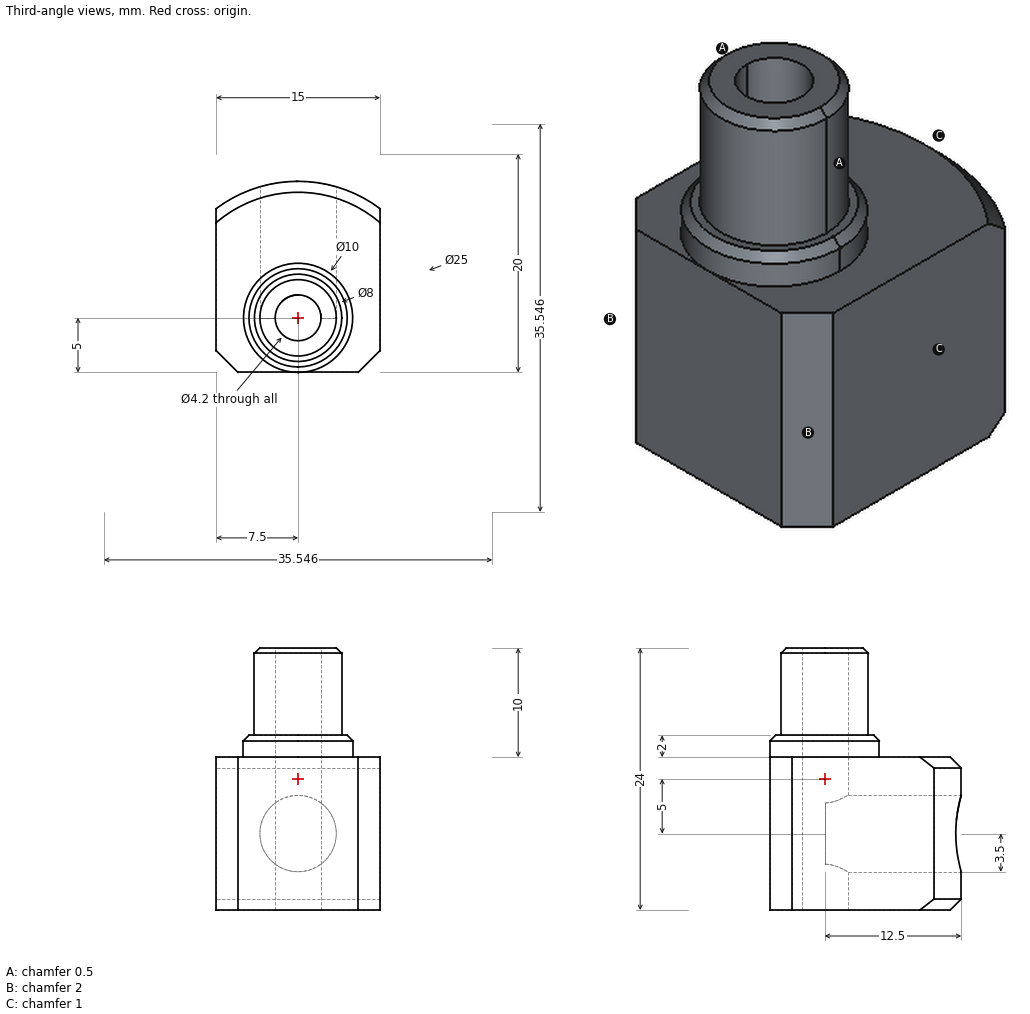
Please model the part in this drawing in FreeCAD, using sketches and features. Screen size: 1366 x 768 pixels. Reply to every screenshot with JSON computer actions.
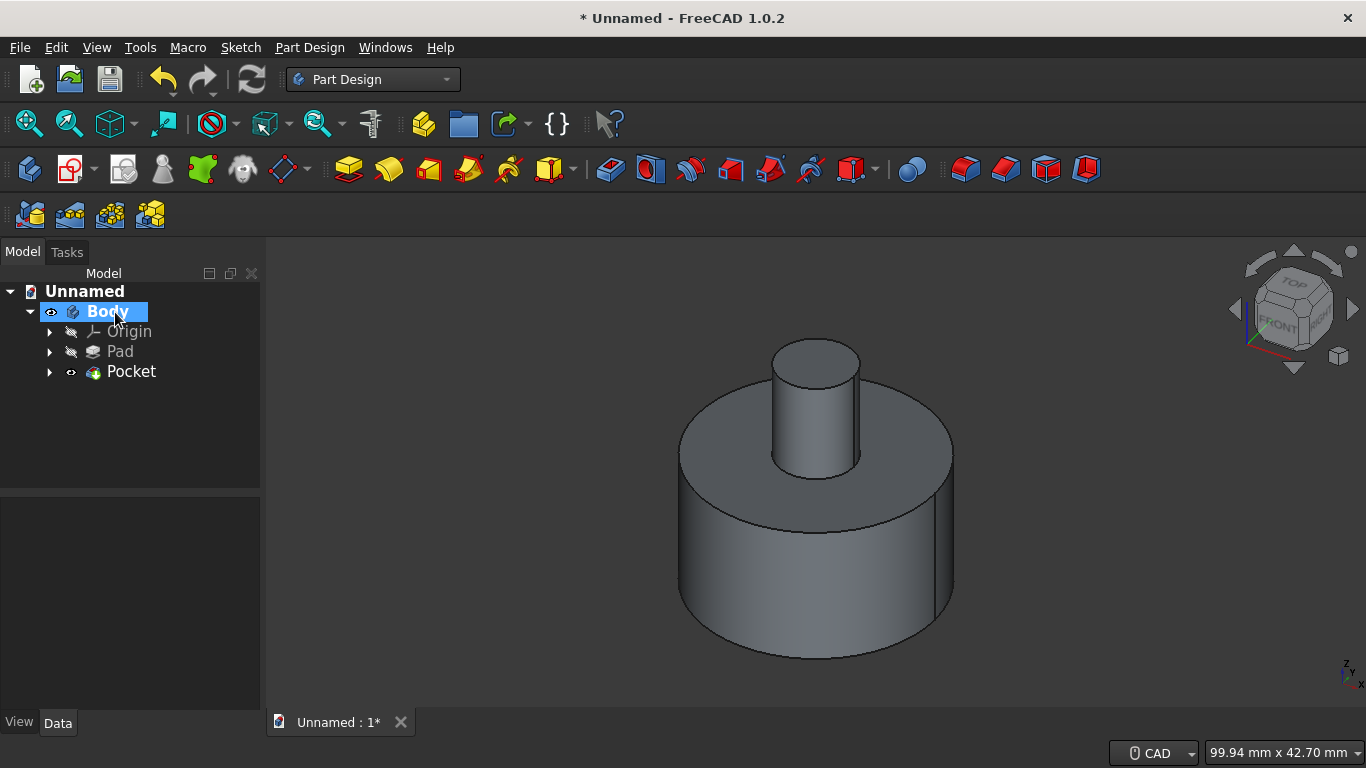
{"action": "key", "text": "5"}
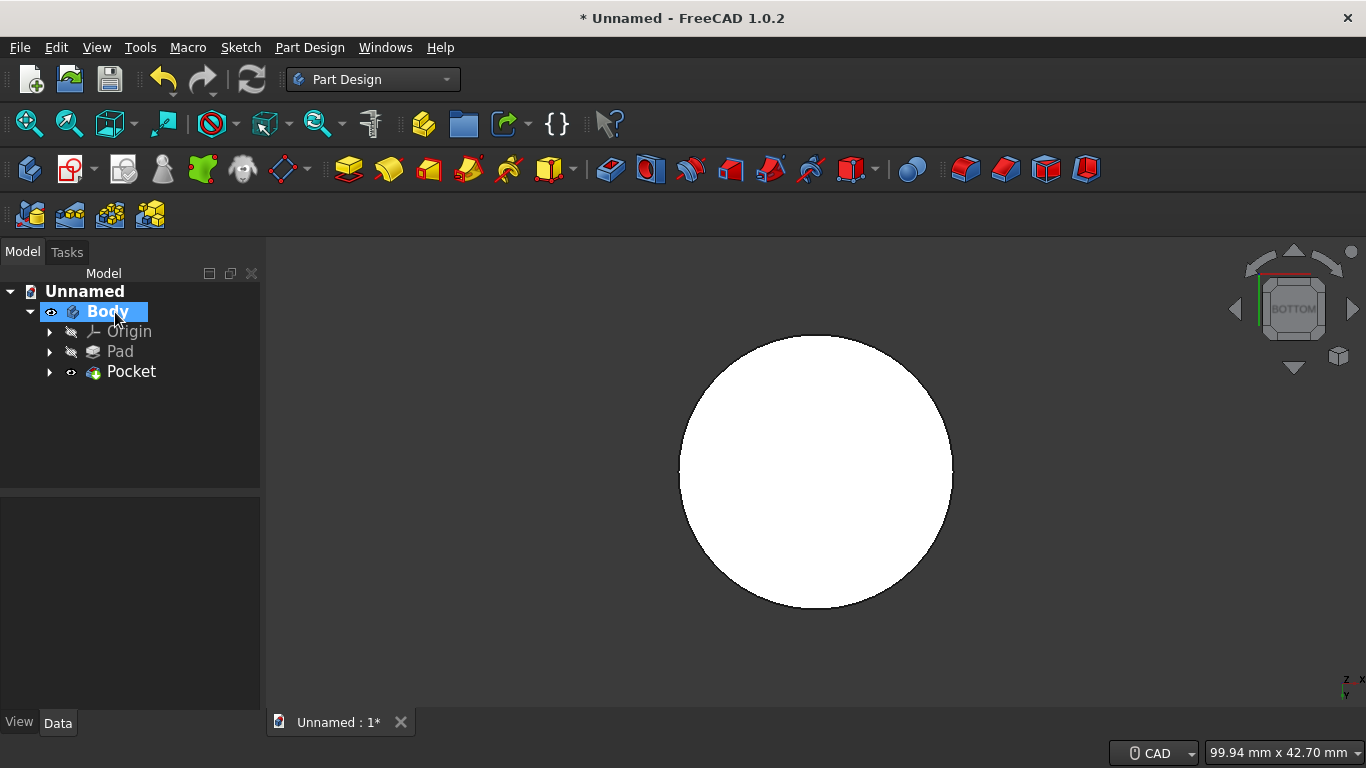
{"action": "left_click", "coordinate": [816, 471]}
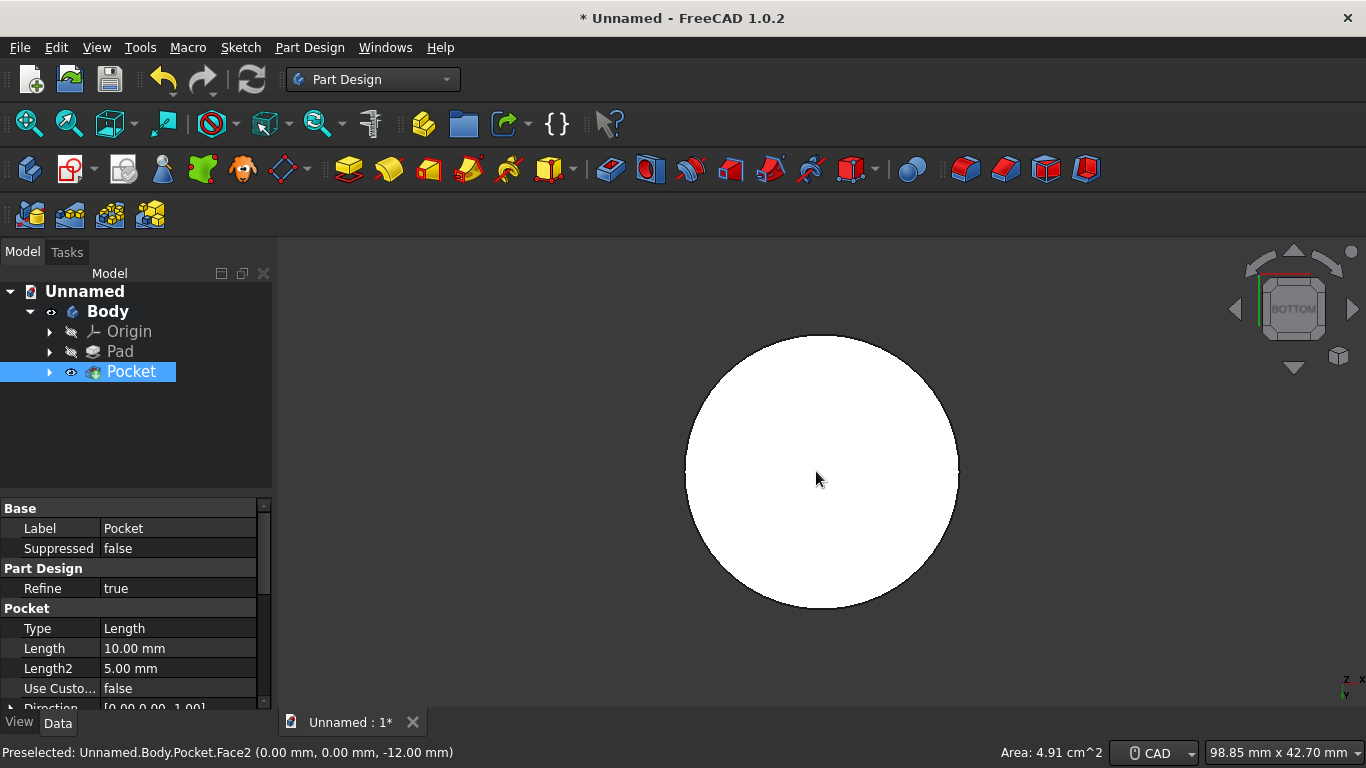
{"action": "left_click", "coordinate": [70, 170]}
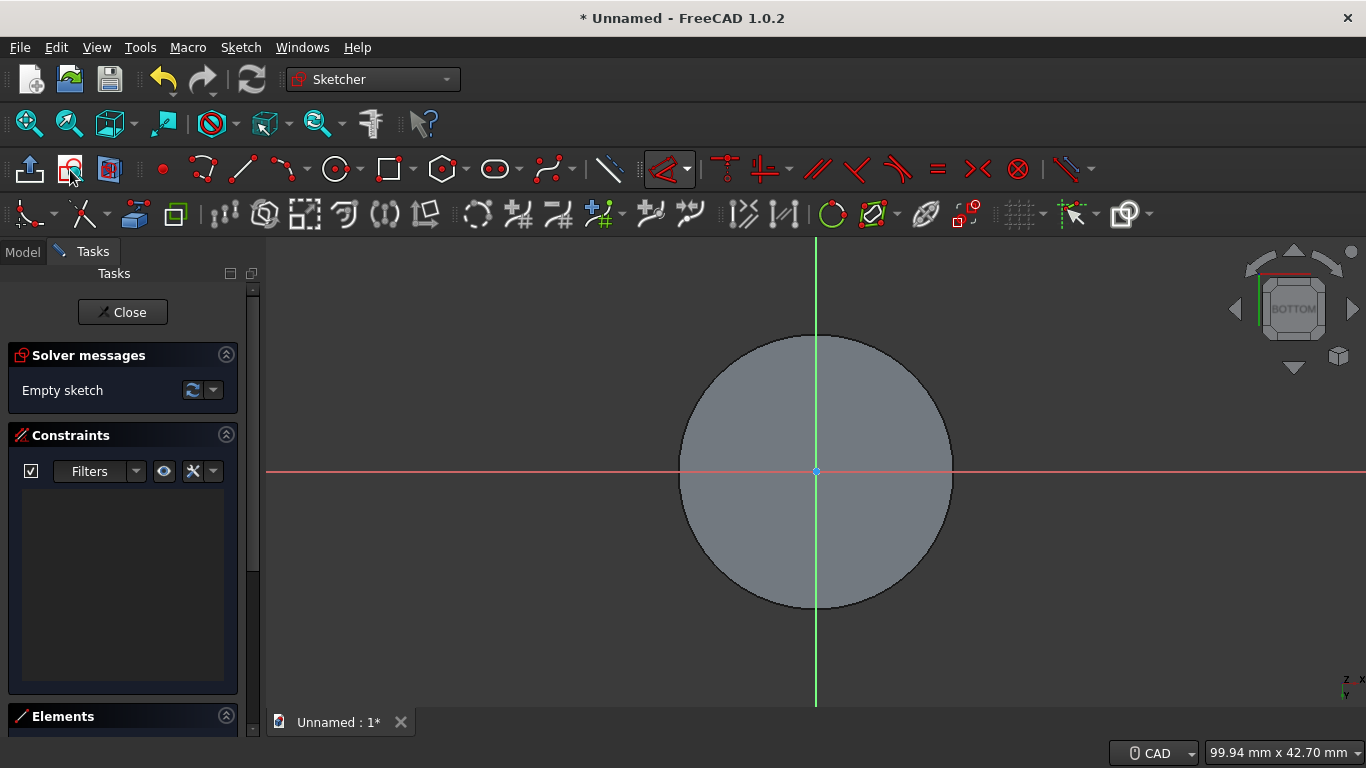
{"action": "scroll", "coordinate": [438, 472], "scroll_direction": "down", "scroll_amount": 1}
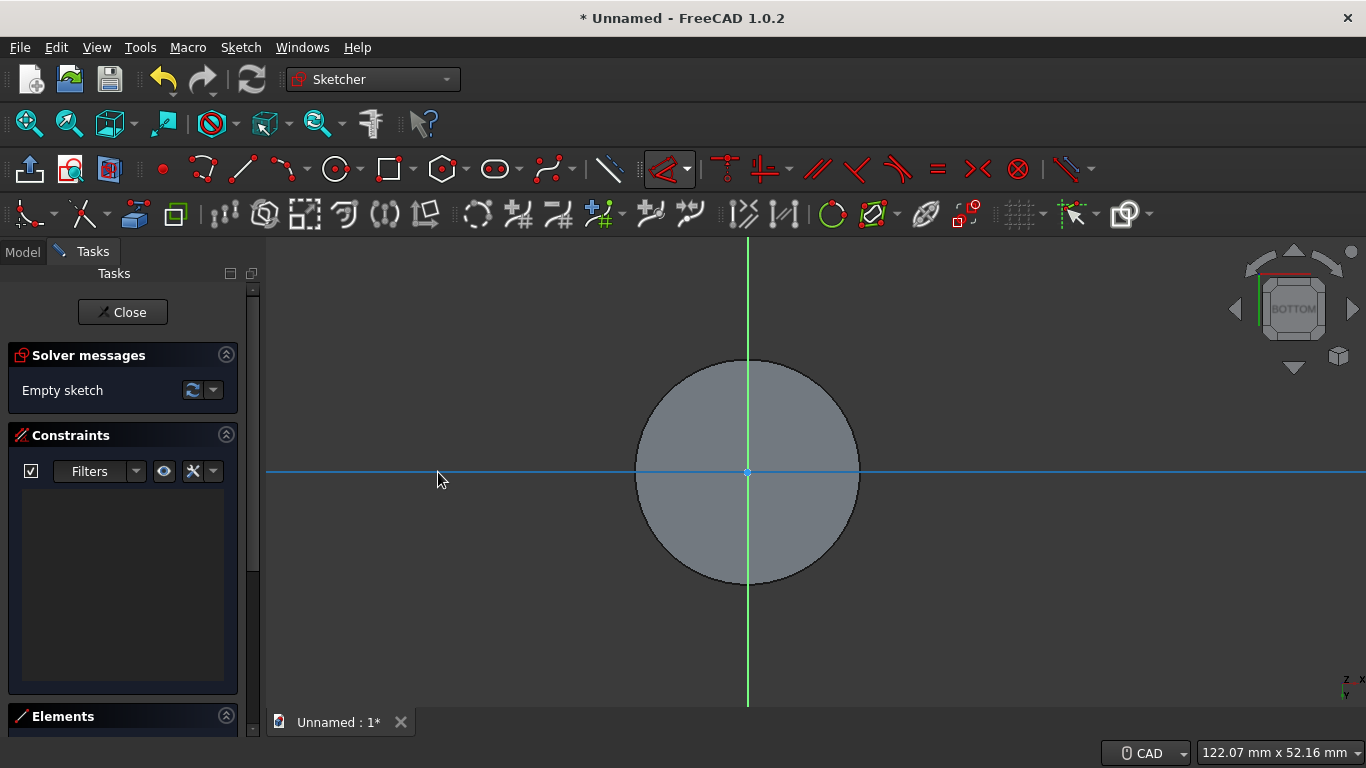
{"action": "key", "text": "g v"}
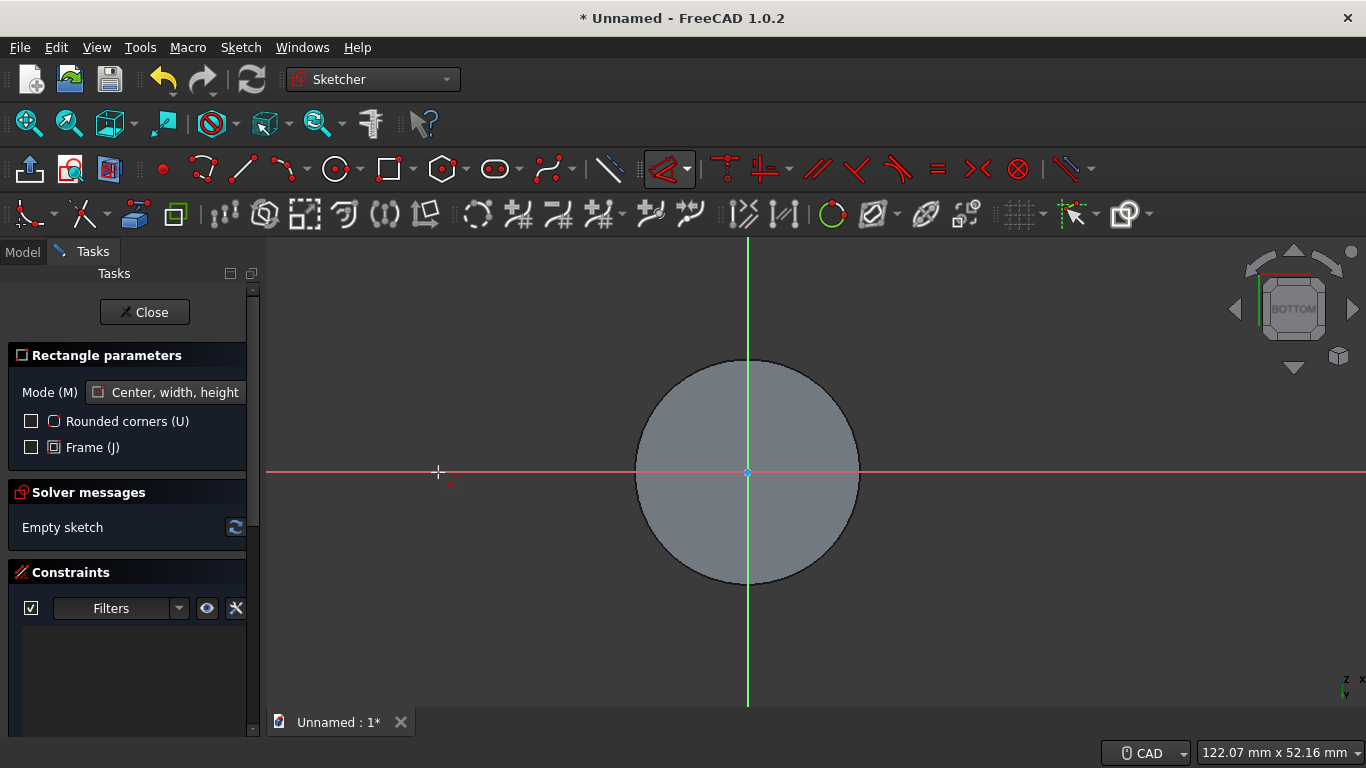
{"action": "left_click", "coordinate": [748, 472]}
{"action": "mouse_move", "coordinate": [908, 312]}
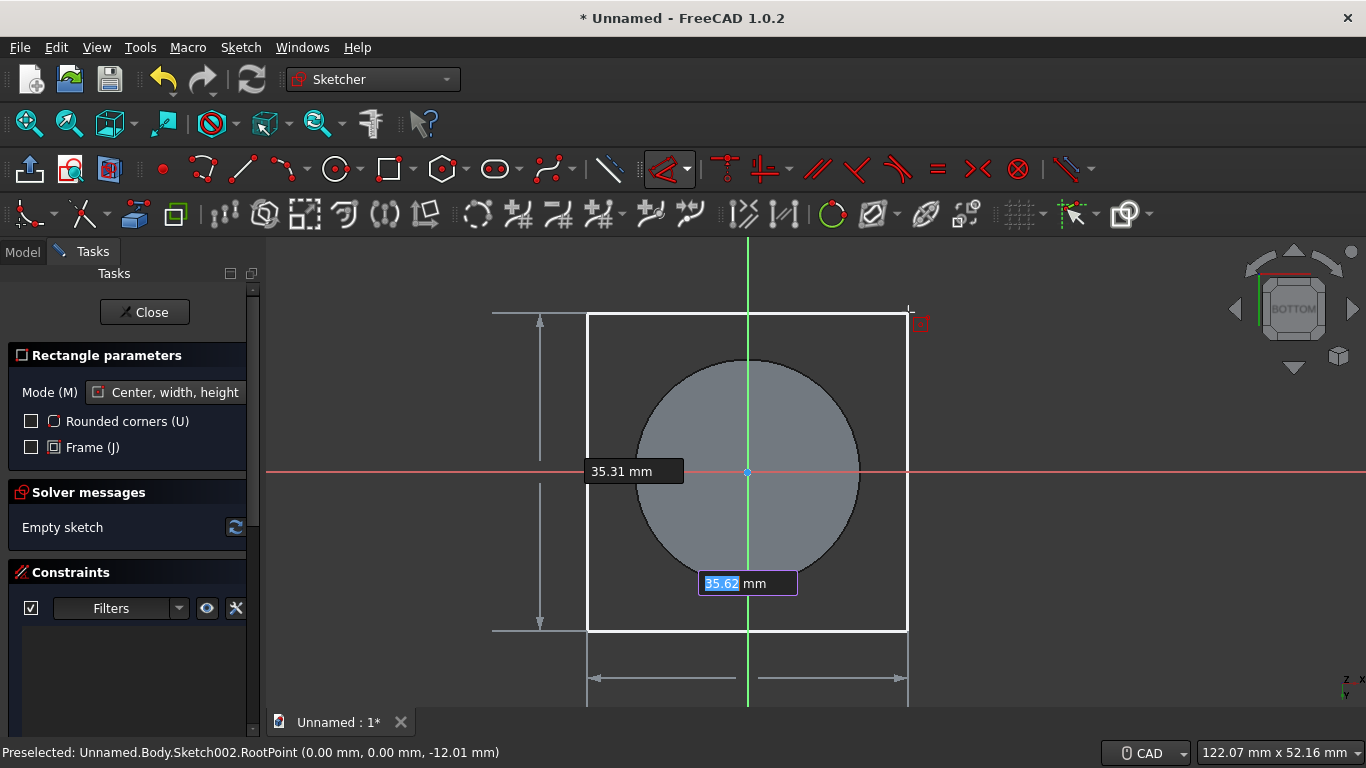
{"action": "type", "text": "35.546"}
{"action": "key", "text": "Tab"}
{"action": "type", "text": "35.546"}
{"action": "key", "text": "Return"}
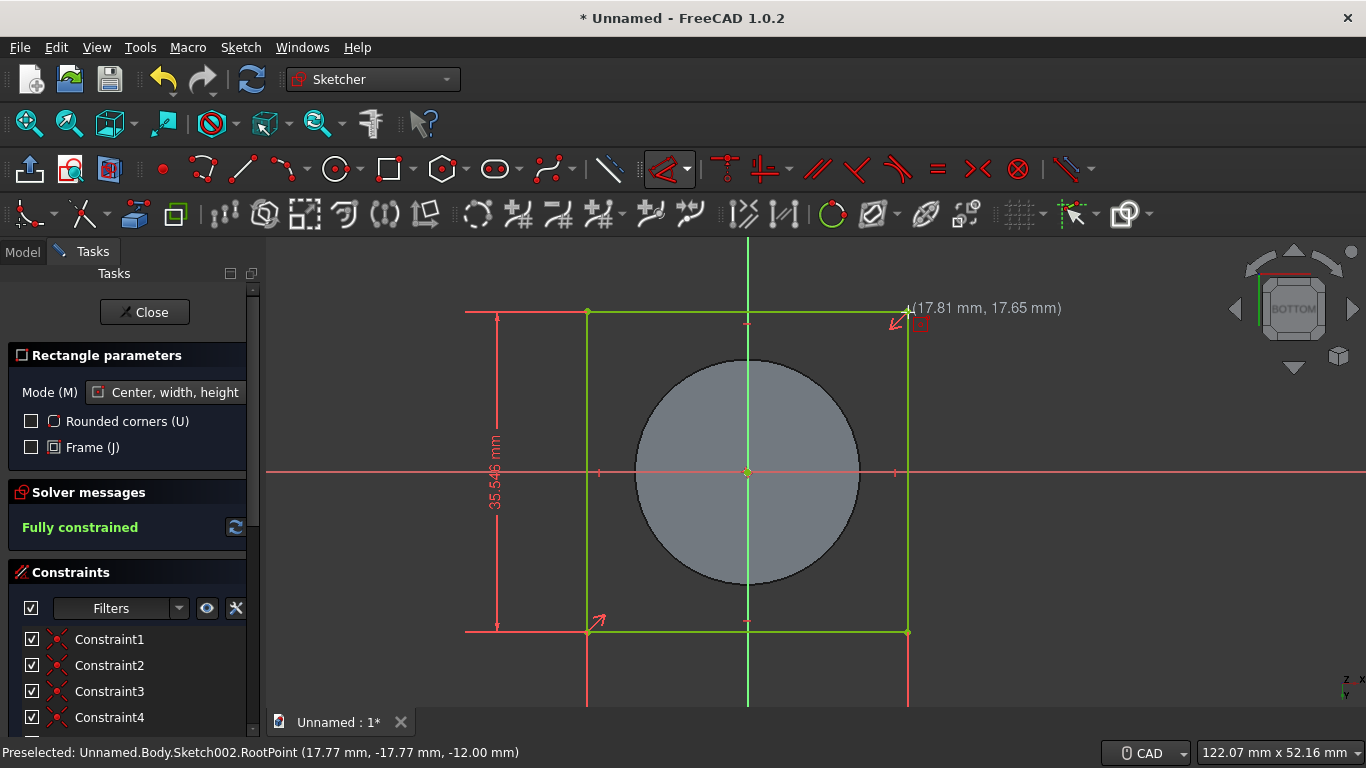
{"action": "left_click", "coordinate": [390, 170]}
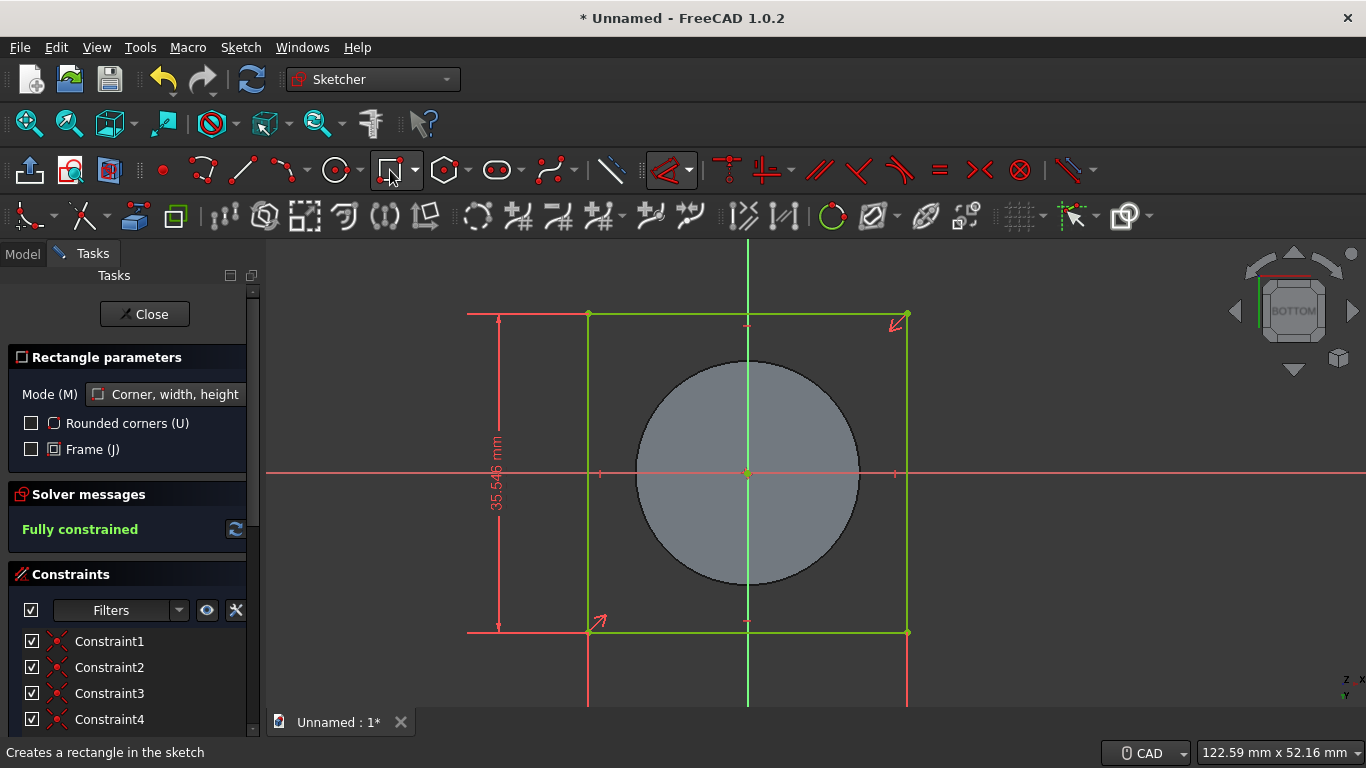
{"action": "left_click", "coordinate": [681, 428]}
{"action": "mouse_move", "coordinate": [815, 608]}